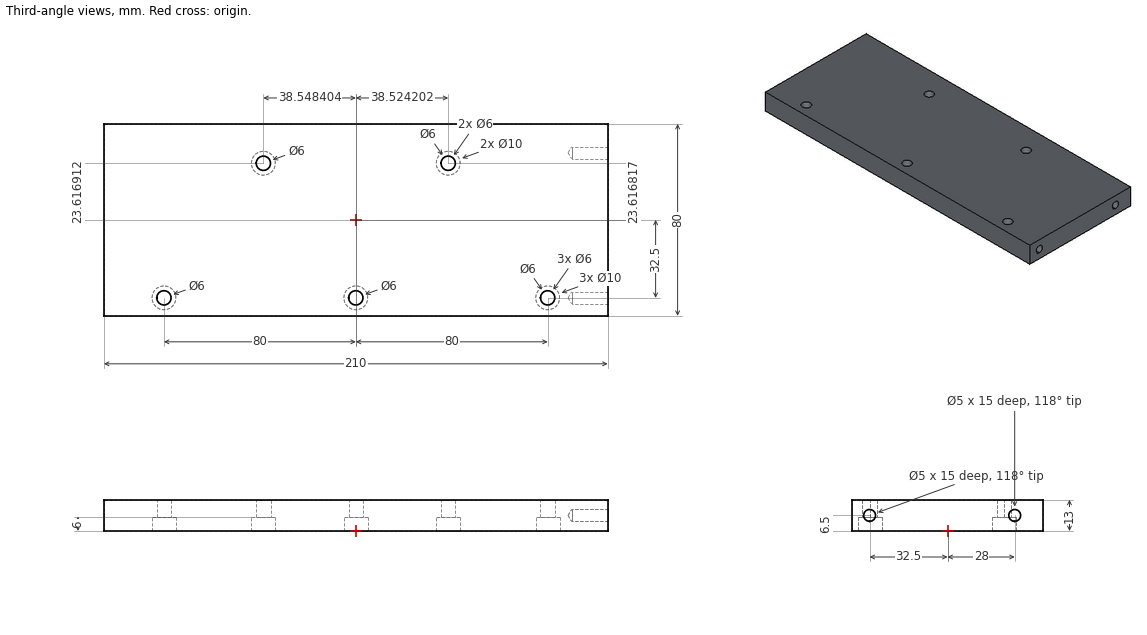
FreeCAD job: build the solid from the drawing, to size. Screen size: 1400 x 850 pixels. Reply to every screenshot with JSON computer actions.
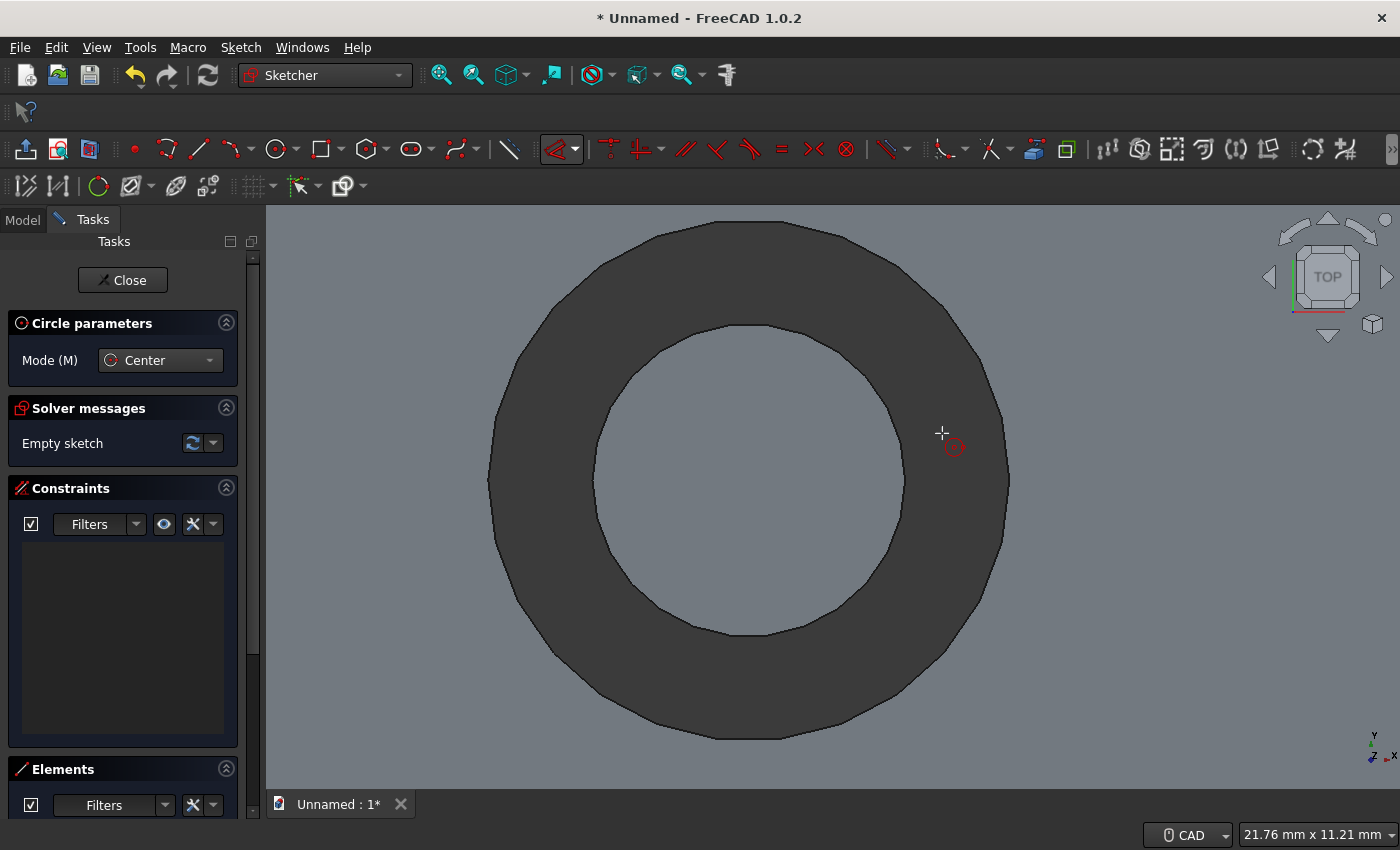
{"action": "left_click", "coordinate": [749, 480]}
{"action": "left_click", "coordinate": [859, 370]}
{"action": "key", "text": "Escape"}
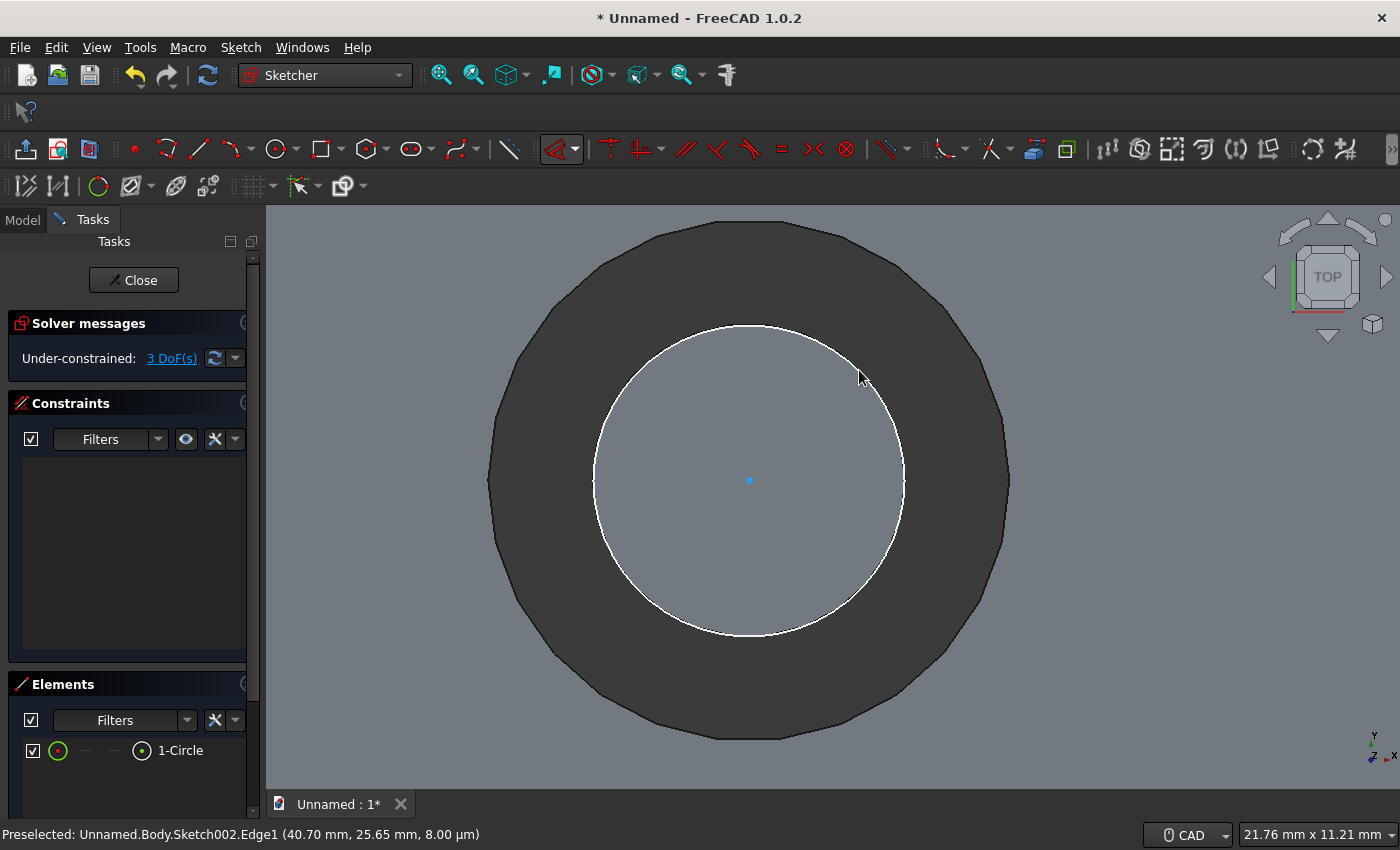
{"action": "left_click", "coordinate": [556, 150]}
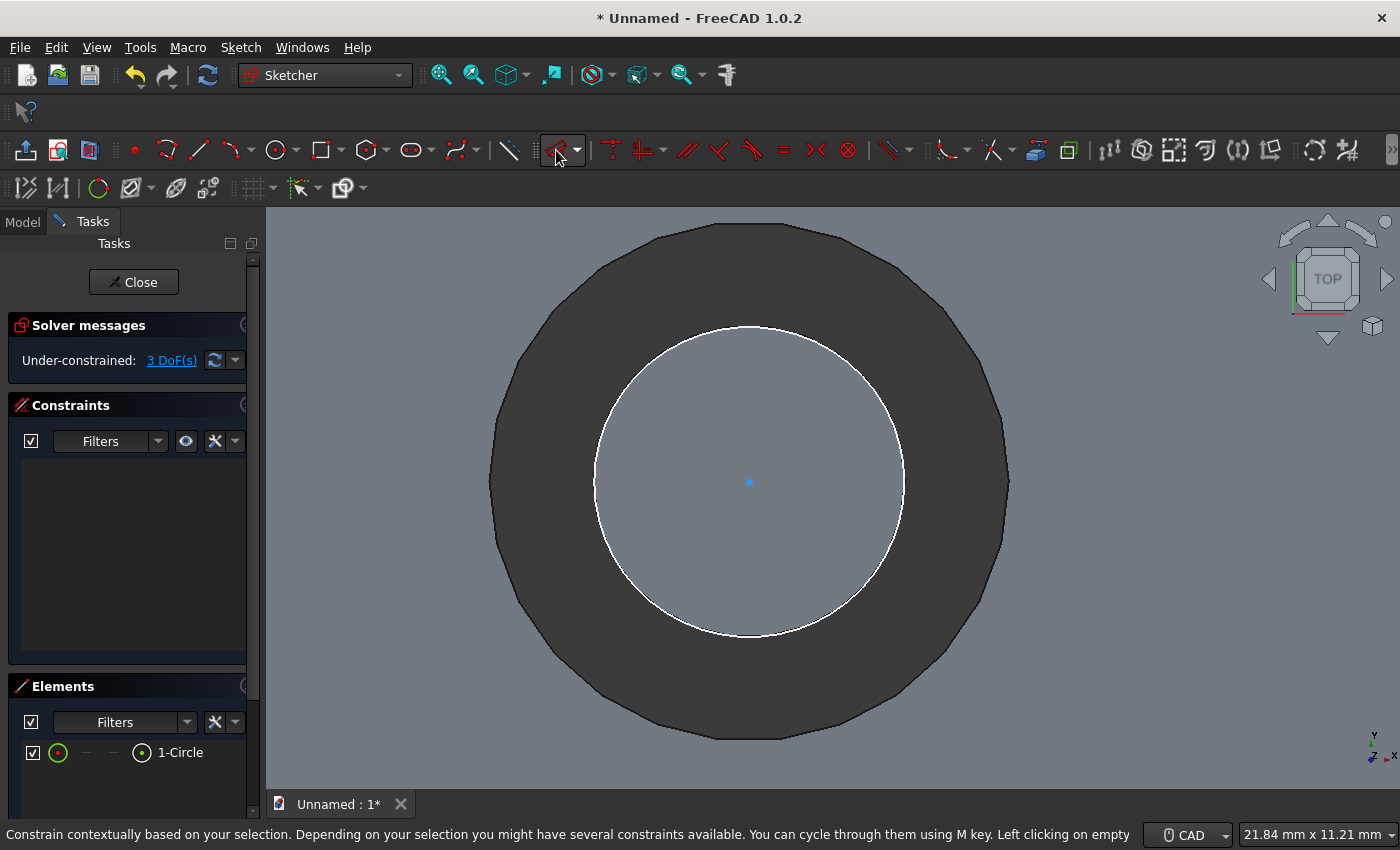
{"action": "left_click", "coordinate": [859, 372]}
{"action": "left_click", "coordinate": [882, 349]}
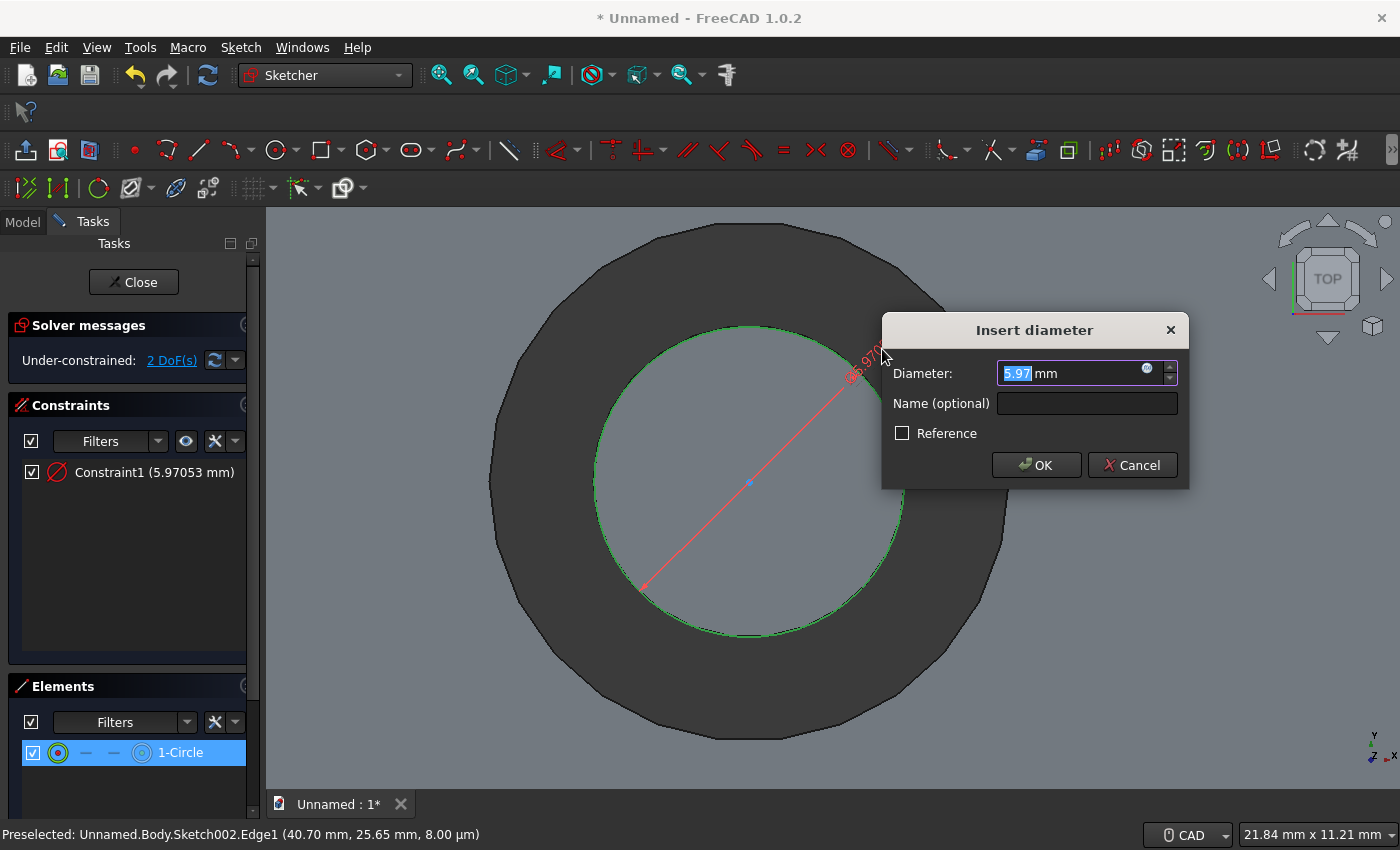
{"action": "type", "text": "6"}
{"action": "key", "text": "Return"}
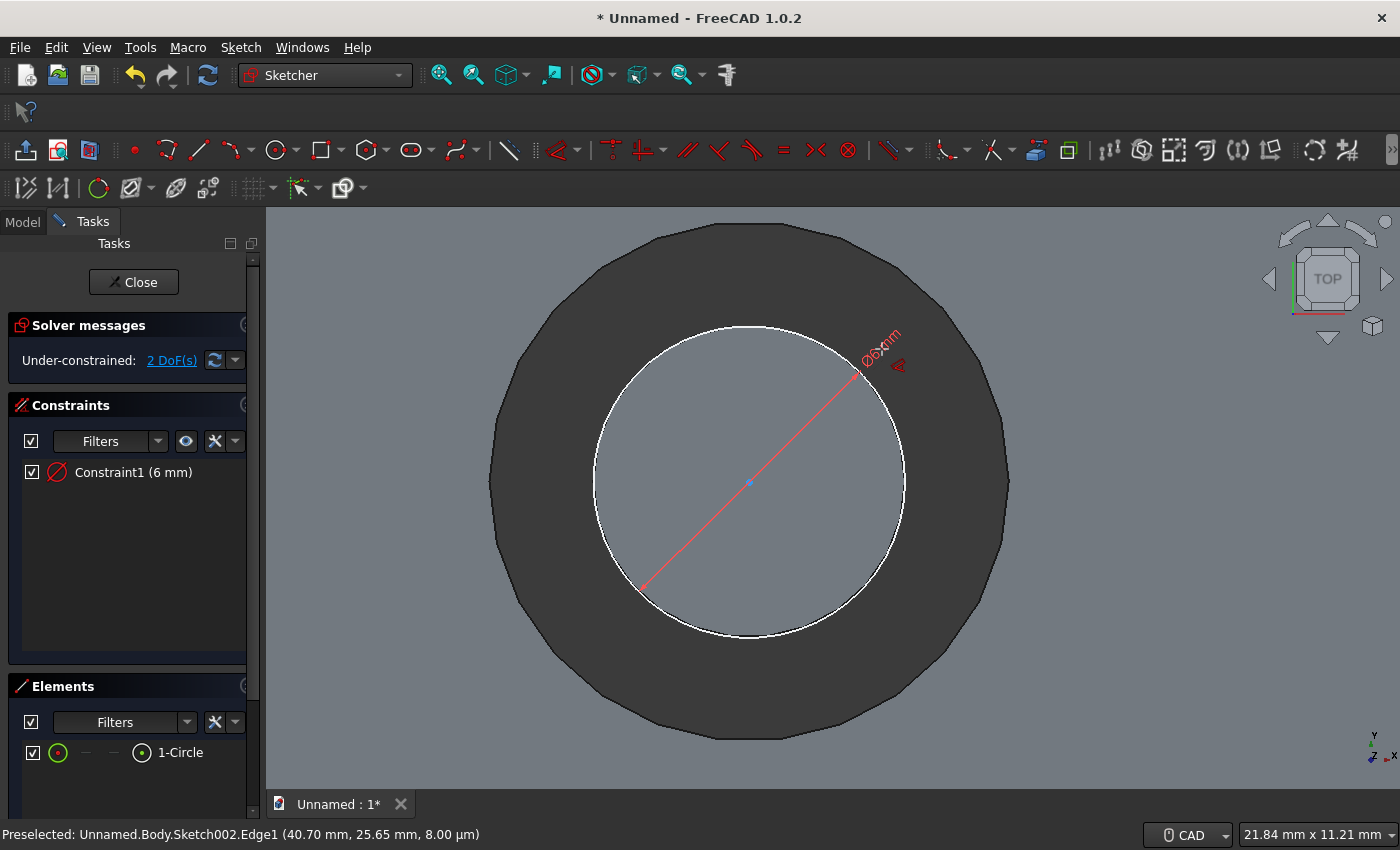
{"action": "left_click", "coordinate": [749, 482]}
{"action": "left_click", "coordinate": [522, 448]}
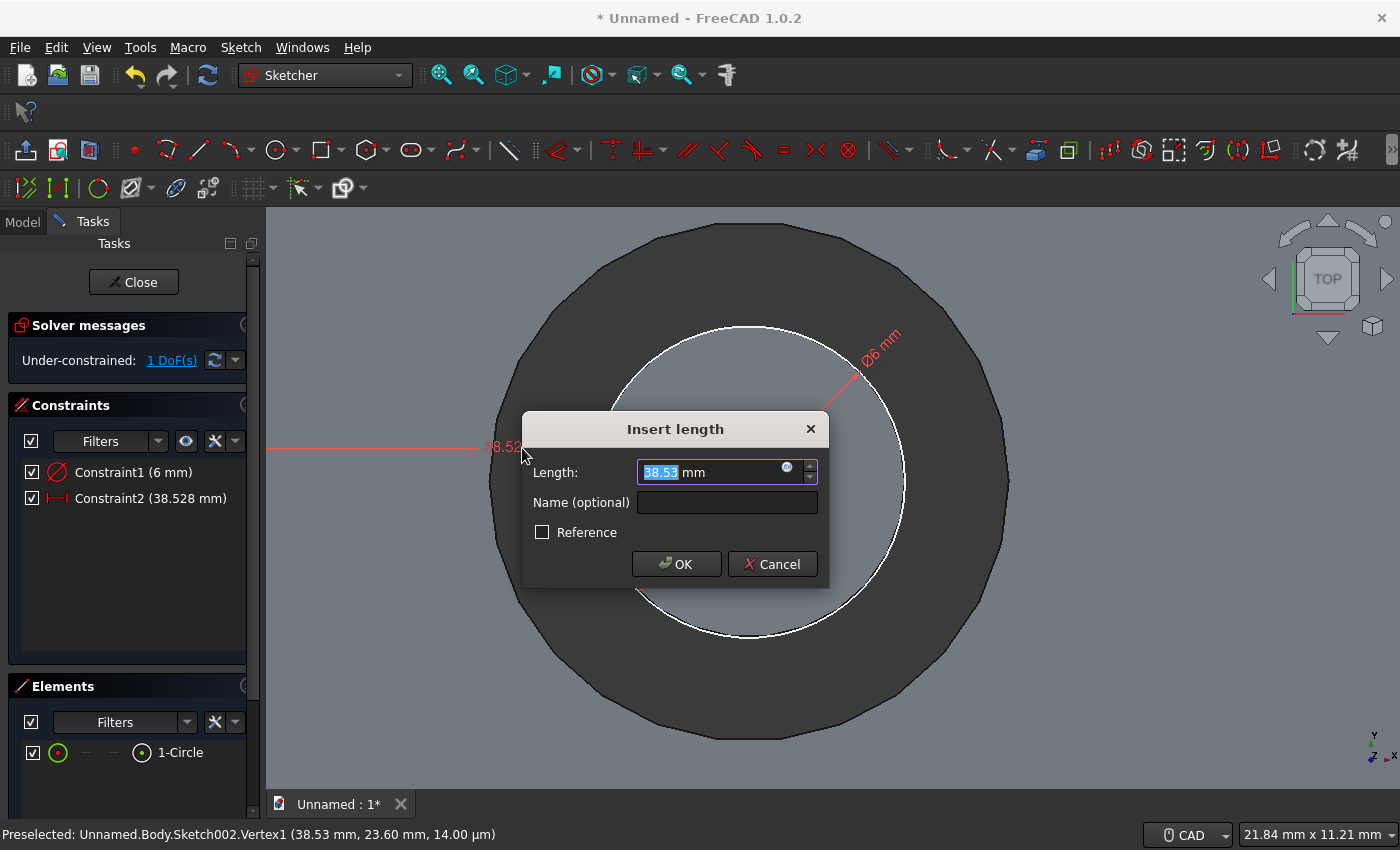
{"action": "type", "text": "38.524202"}
{"action": "key", "text": "Return"}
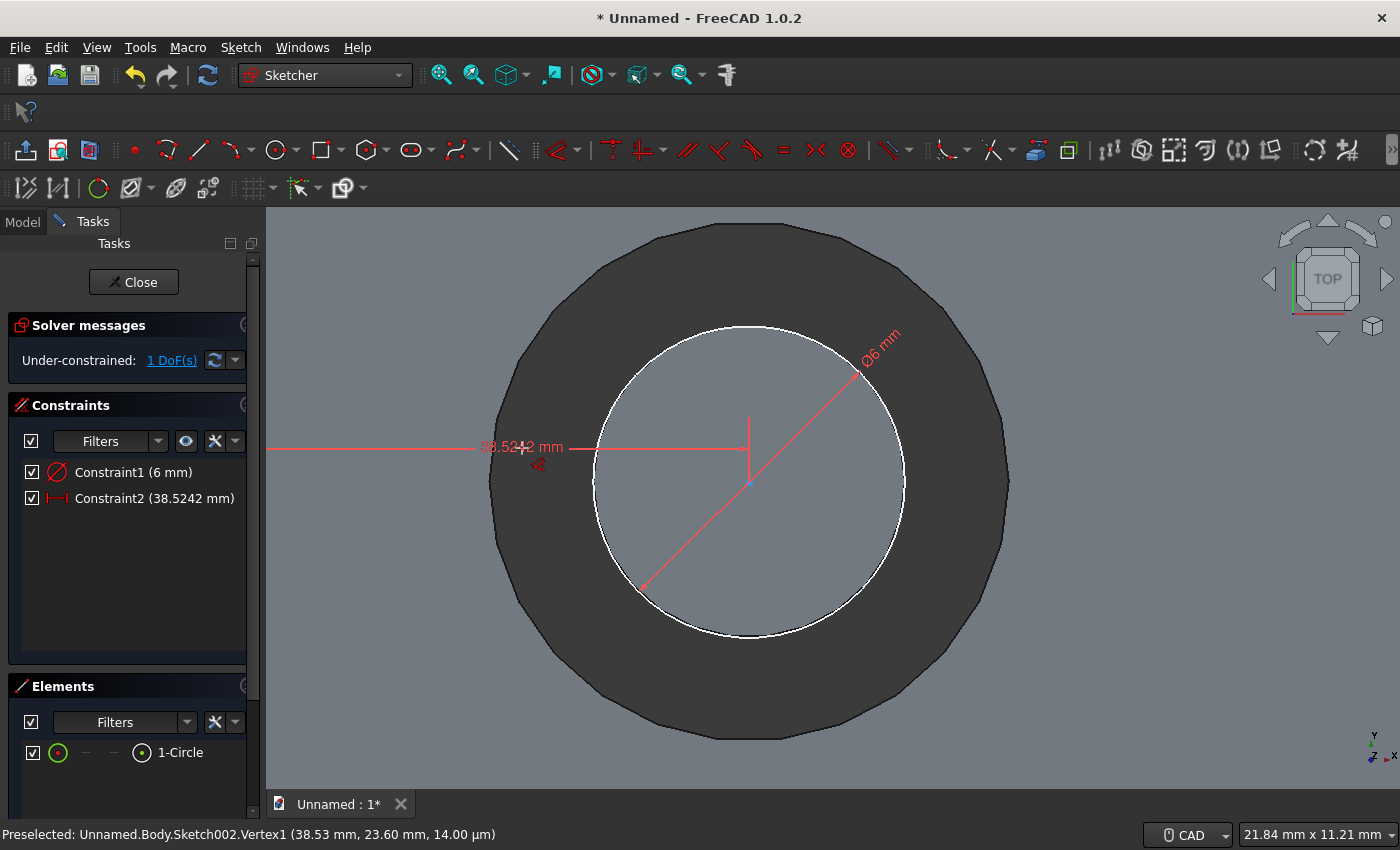
{"action": "left_click", "coordinate": [749, 482]}
{"action": "left_click", "coordinate": [783, 557]}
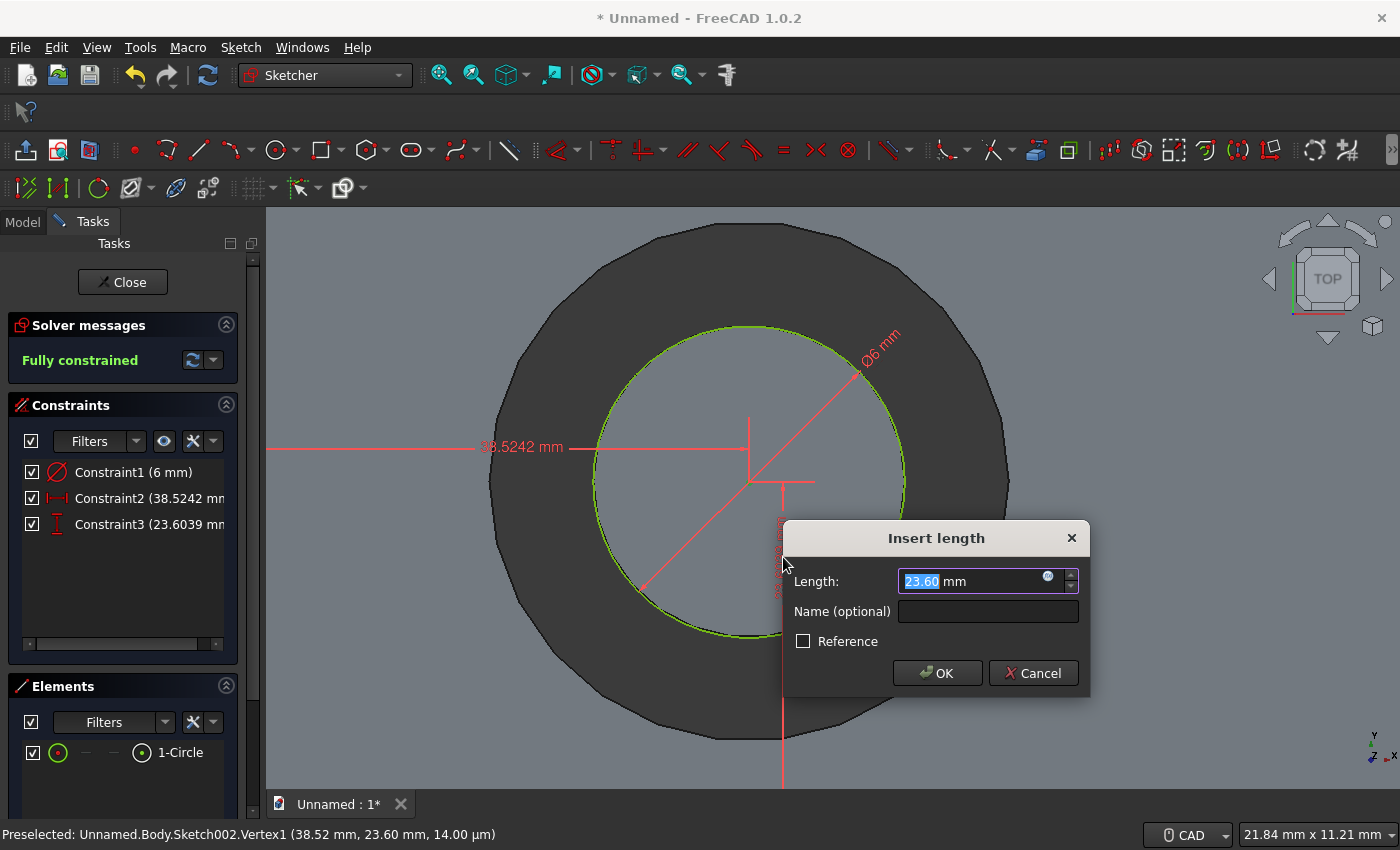
{"action": "type", "text": "23.616817"}
{"action": "key", "text": "Return"}
{"action": "key", "text": "Escape"}